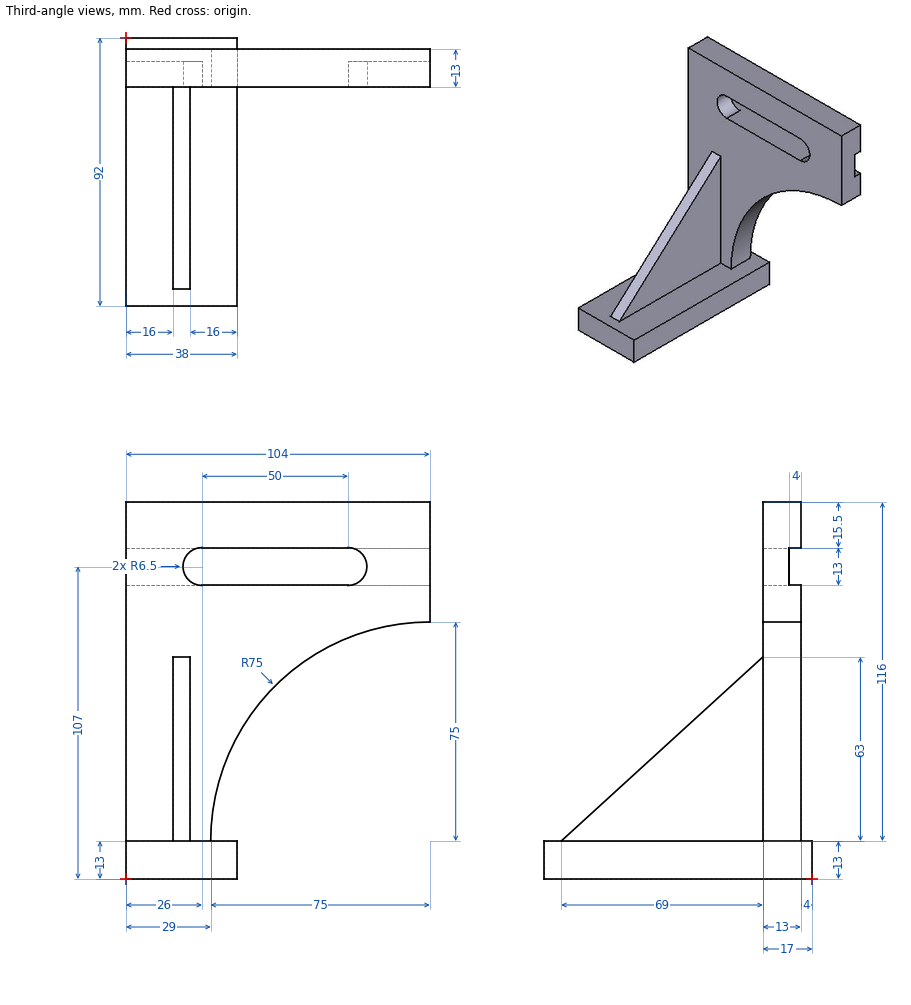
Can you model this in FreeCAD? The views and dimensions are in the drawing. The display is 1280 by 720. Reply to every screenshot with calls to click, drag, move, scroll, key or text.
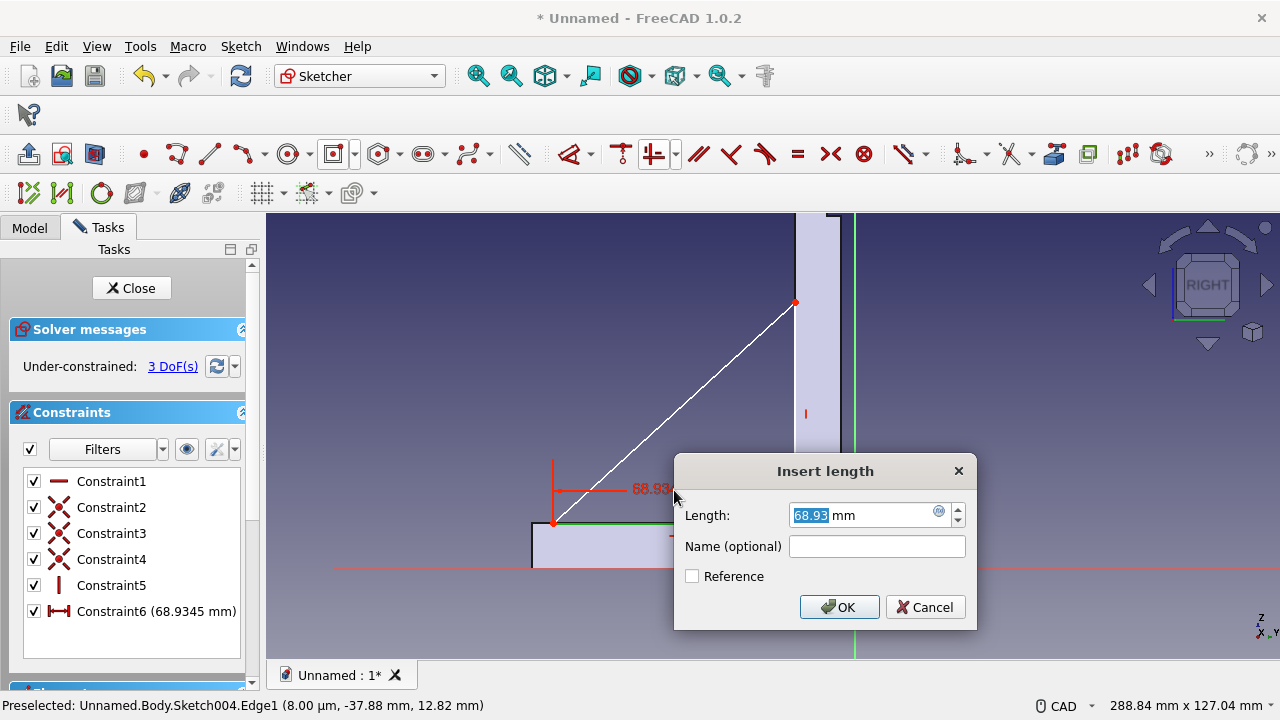
text(69)
key(Return)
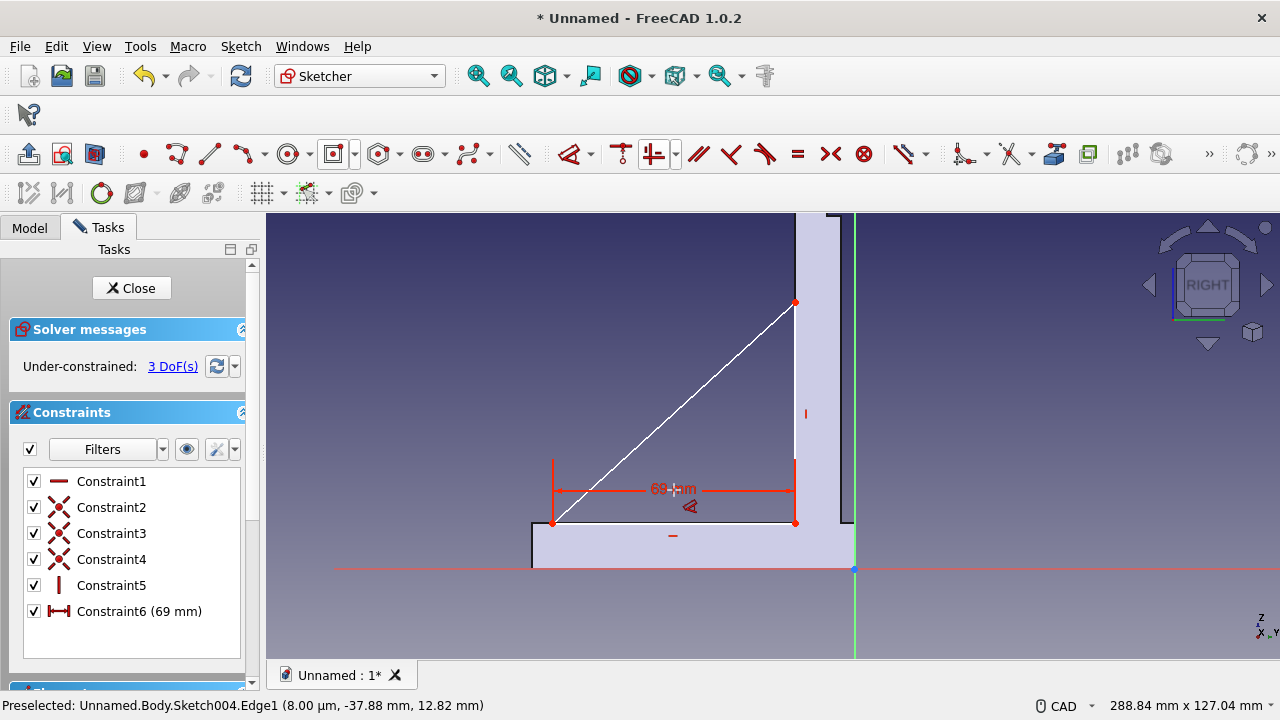
click(795, 369)
click(829, 414)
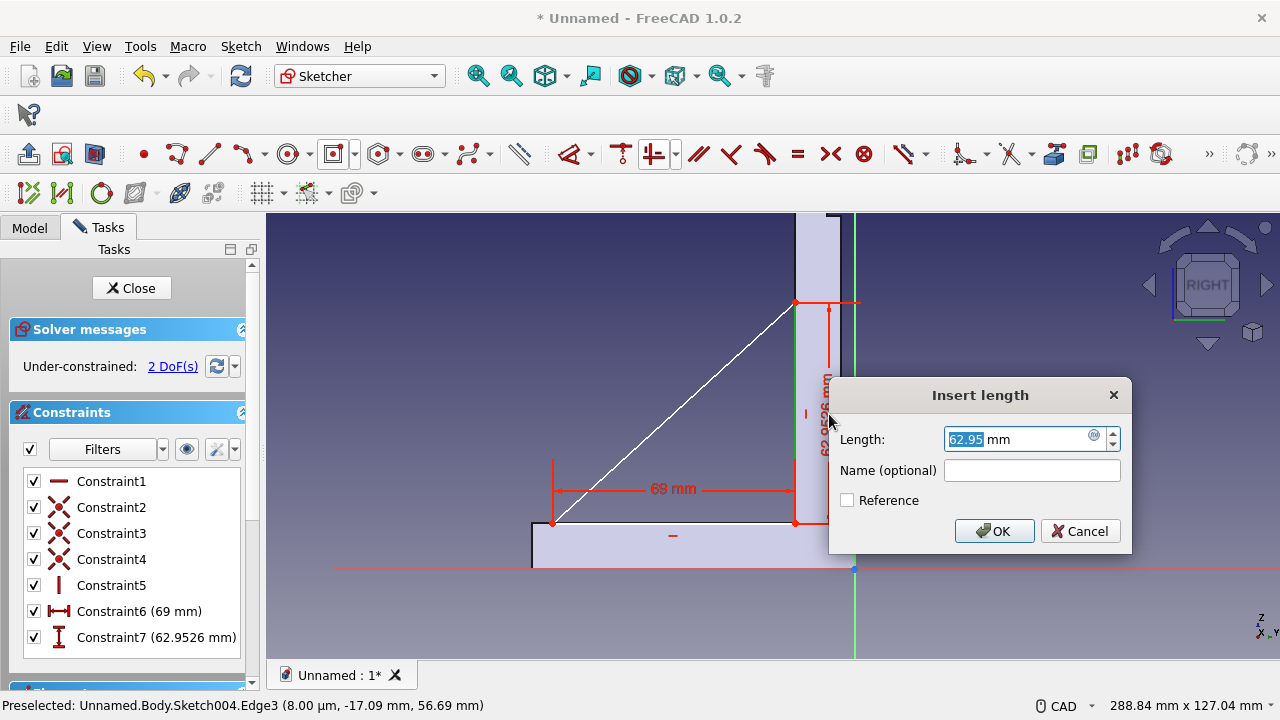
text(63)
key(Return)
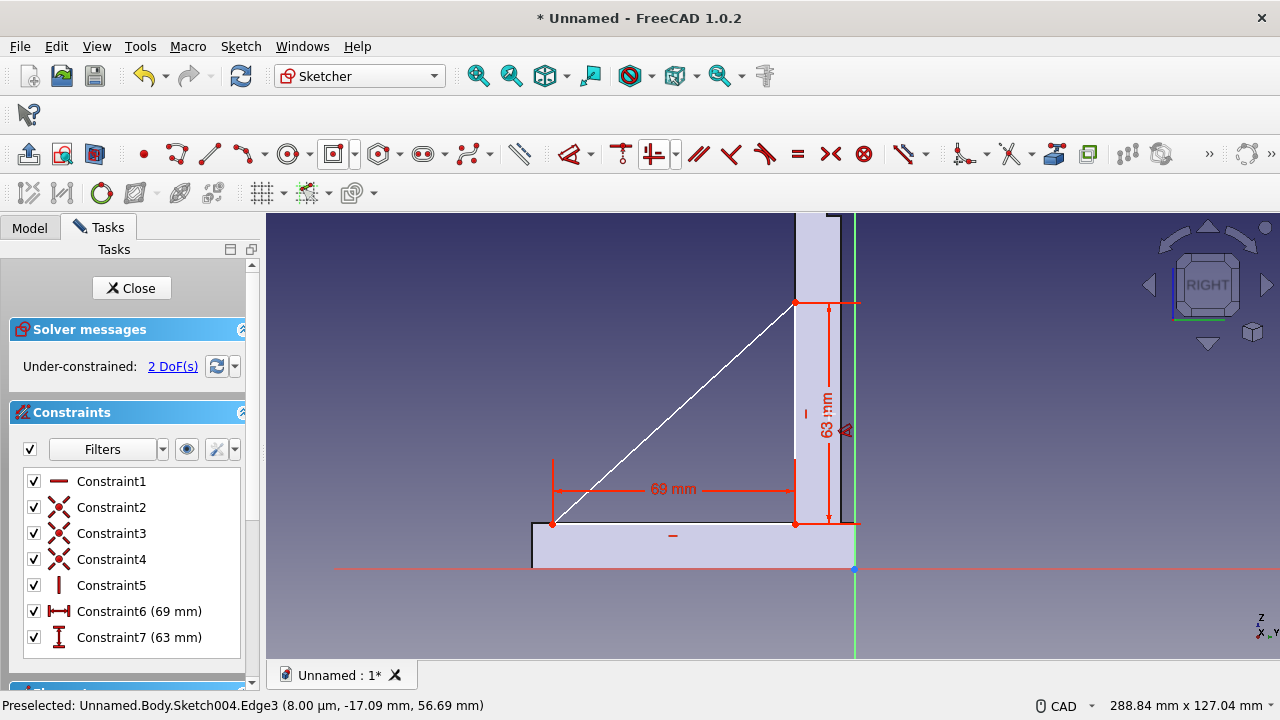
click(795, 524)
click(825, 603)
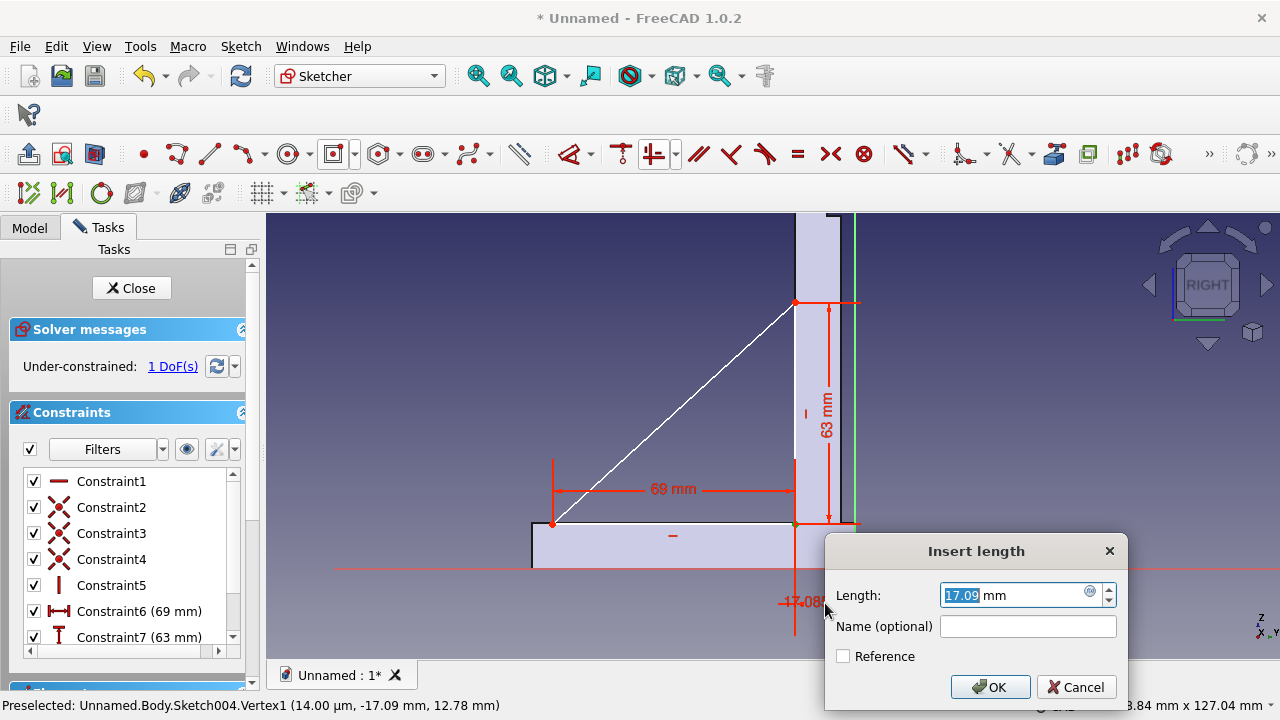
text(17)
key(Return)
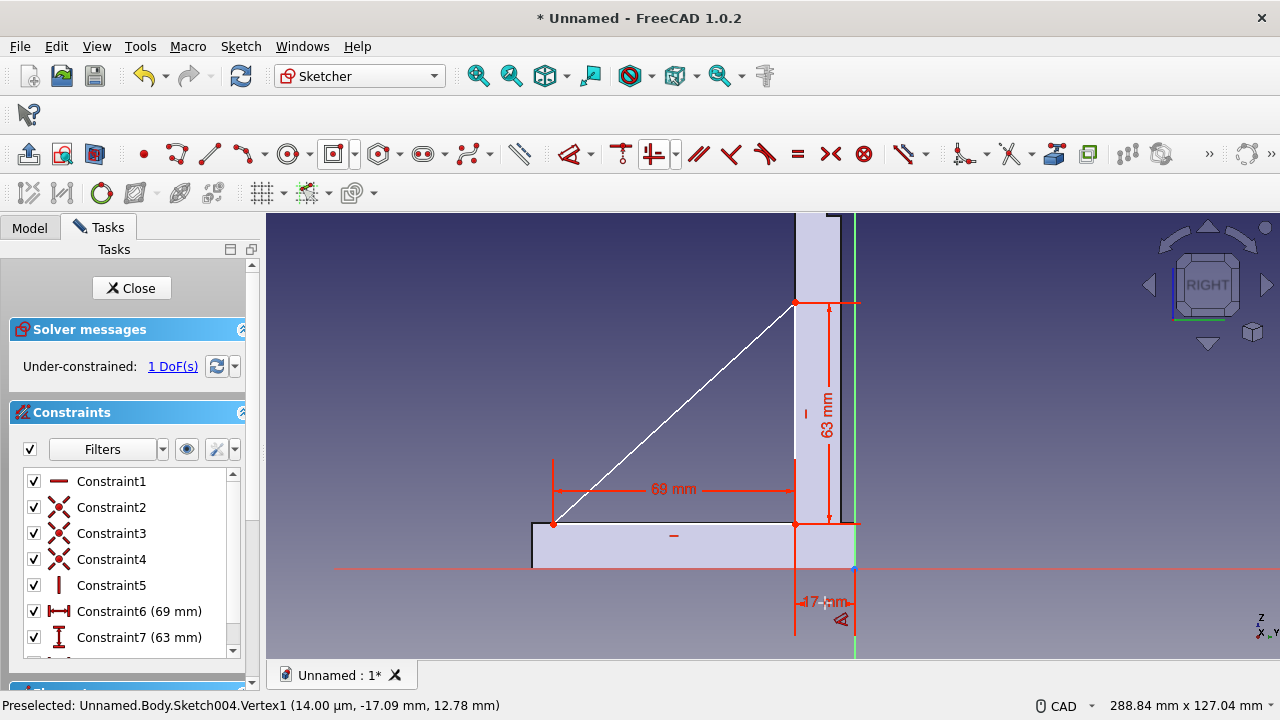
click(795, 524)
click(889, 547)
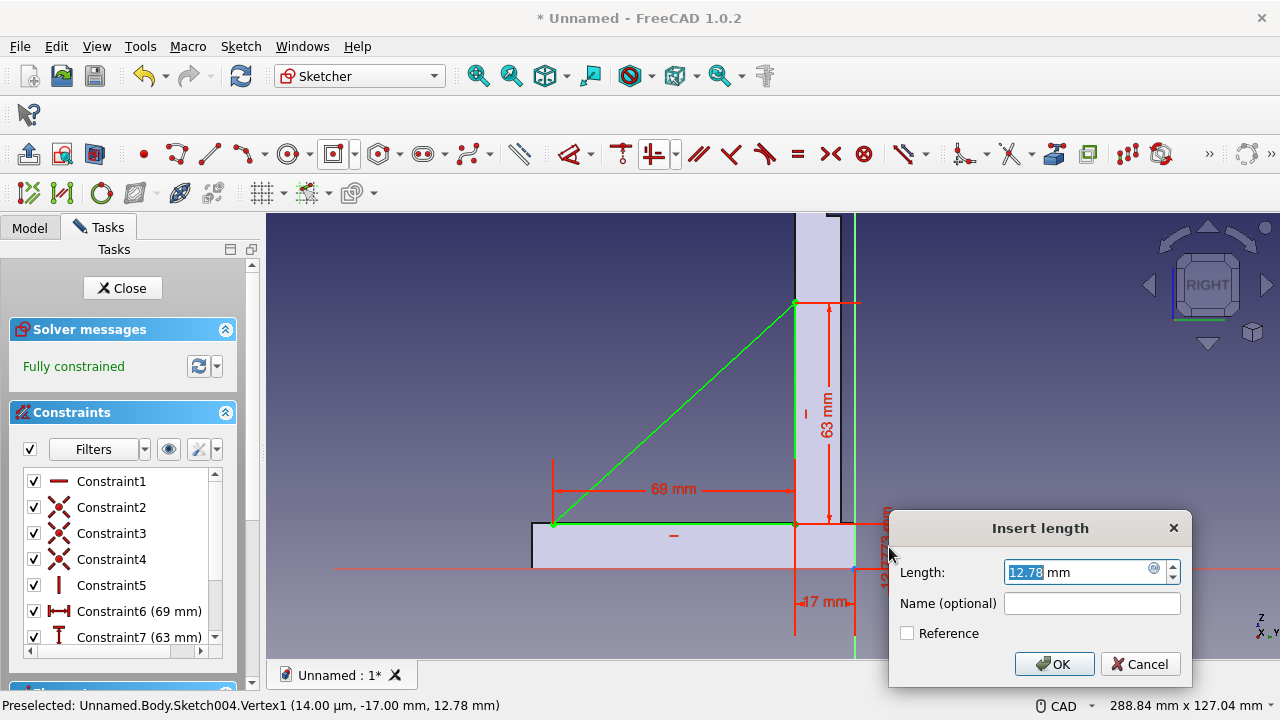
text(13)
key(Return)
key(Escape)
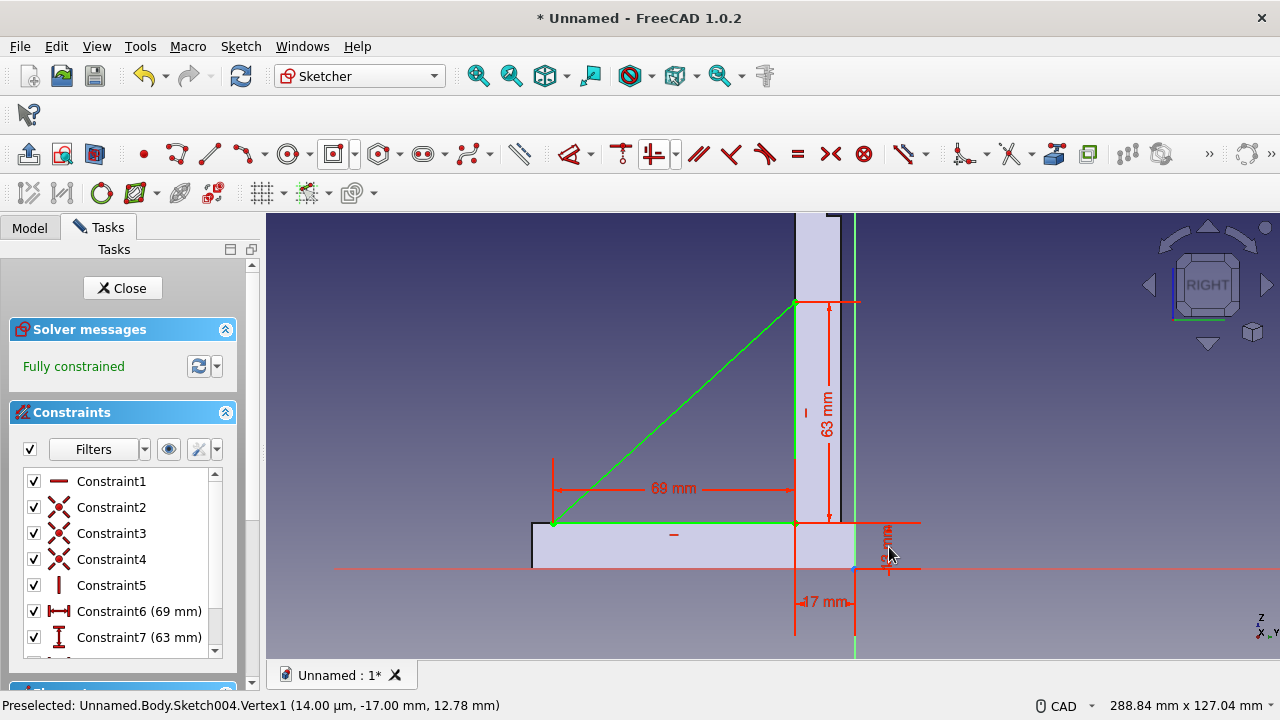
click(123, 288)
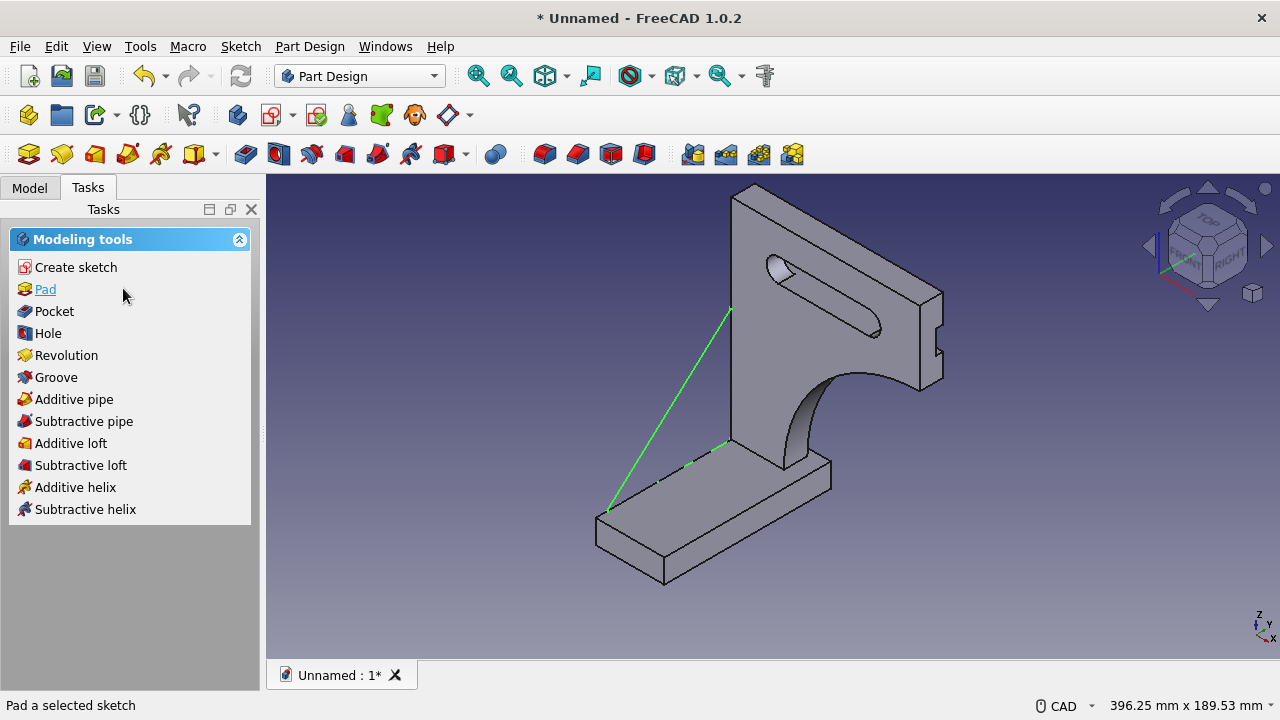
click(29, 154)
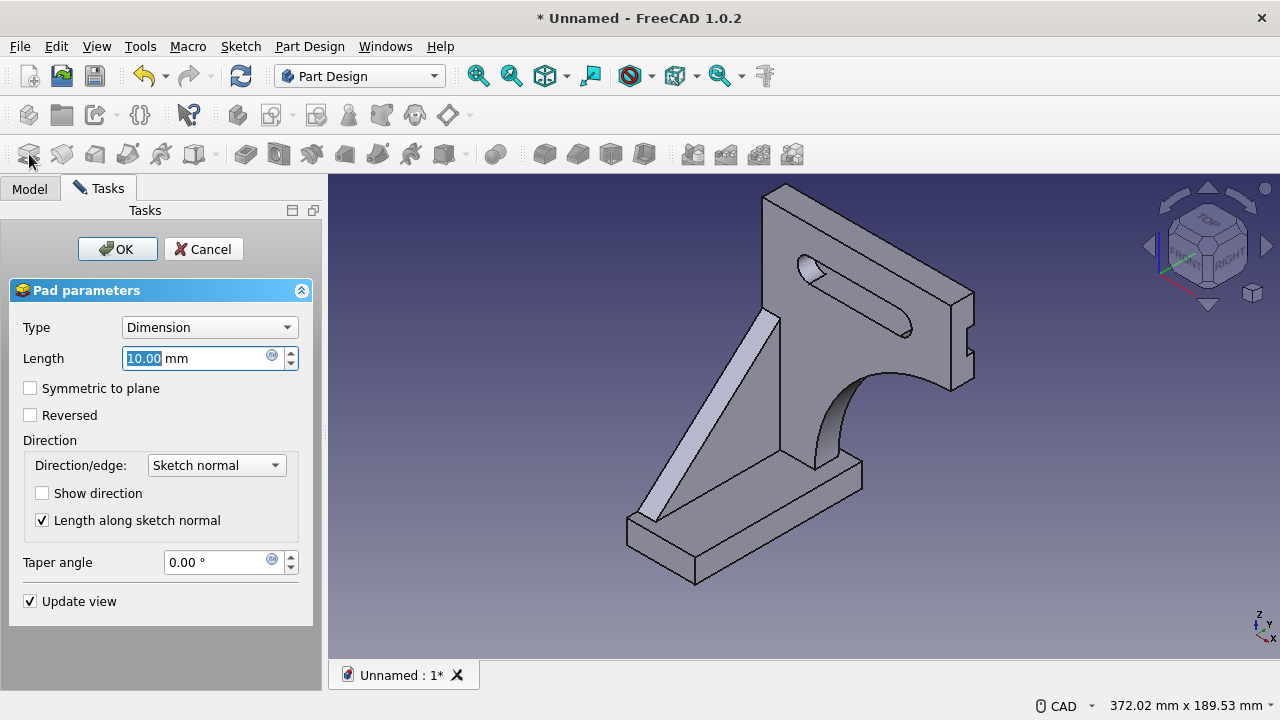
text(38)
key(Tab)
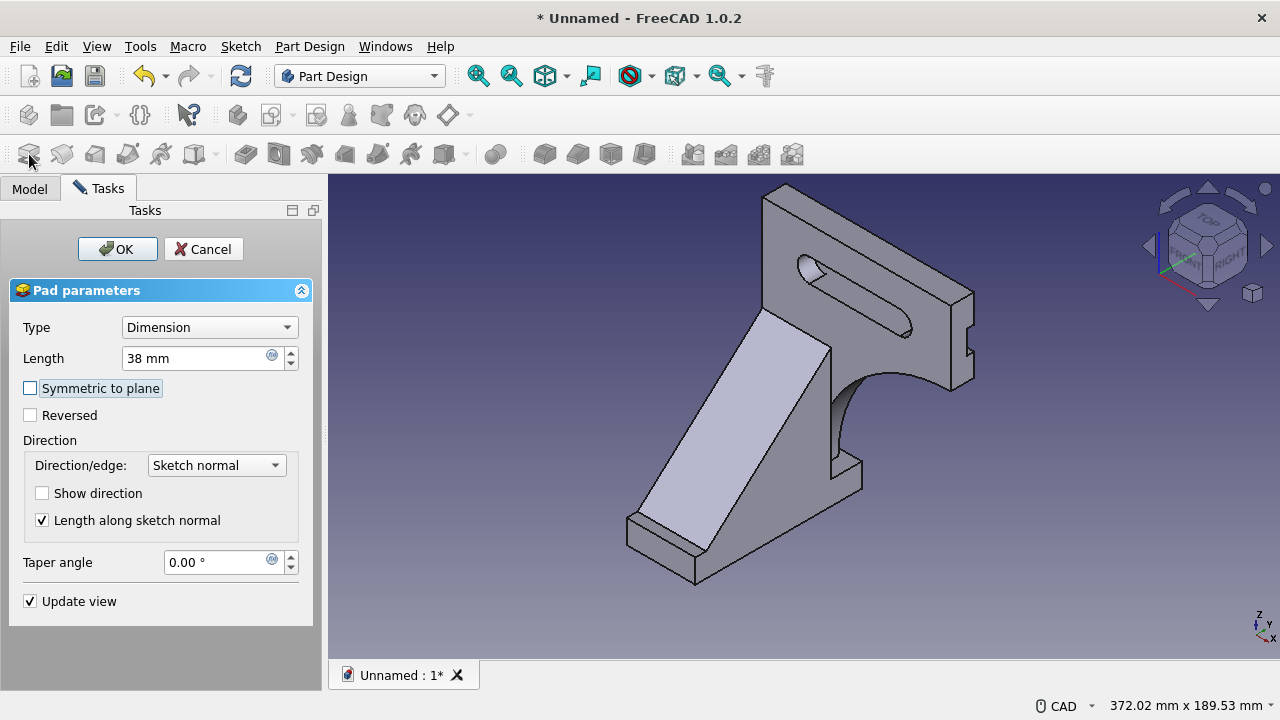
click(118, 249)